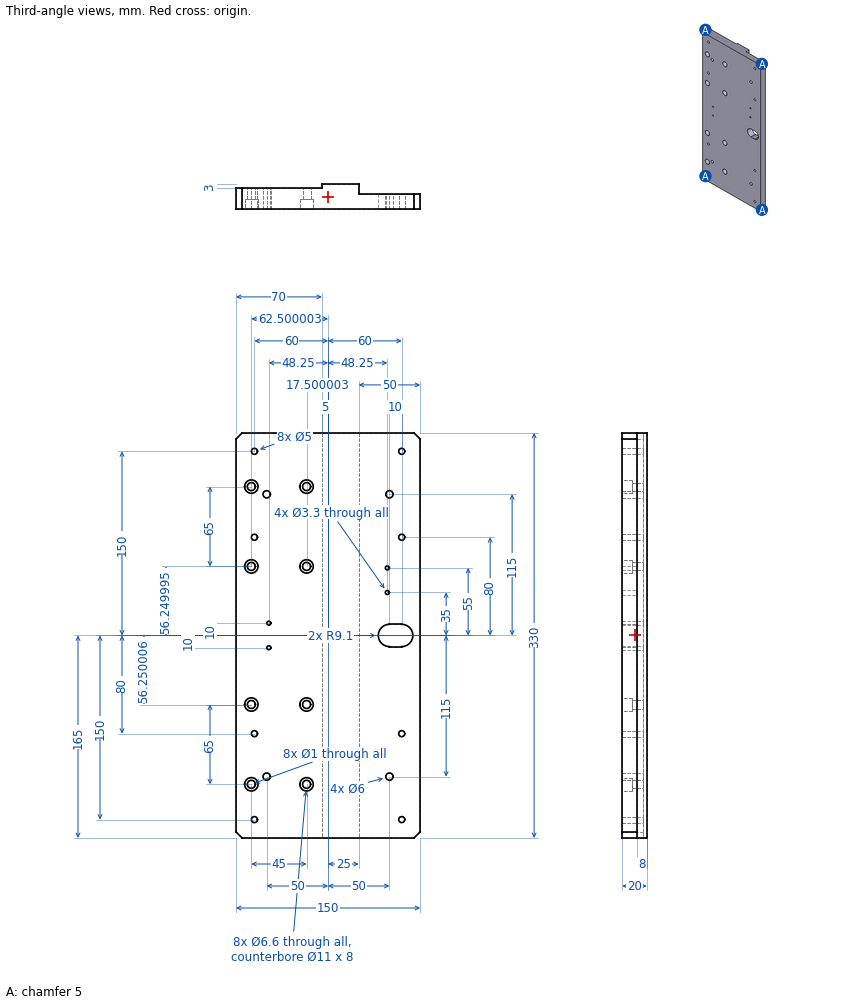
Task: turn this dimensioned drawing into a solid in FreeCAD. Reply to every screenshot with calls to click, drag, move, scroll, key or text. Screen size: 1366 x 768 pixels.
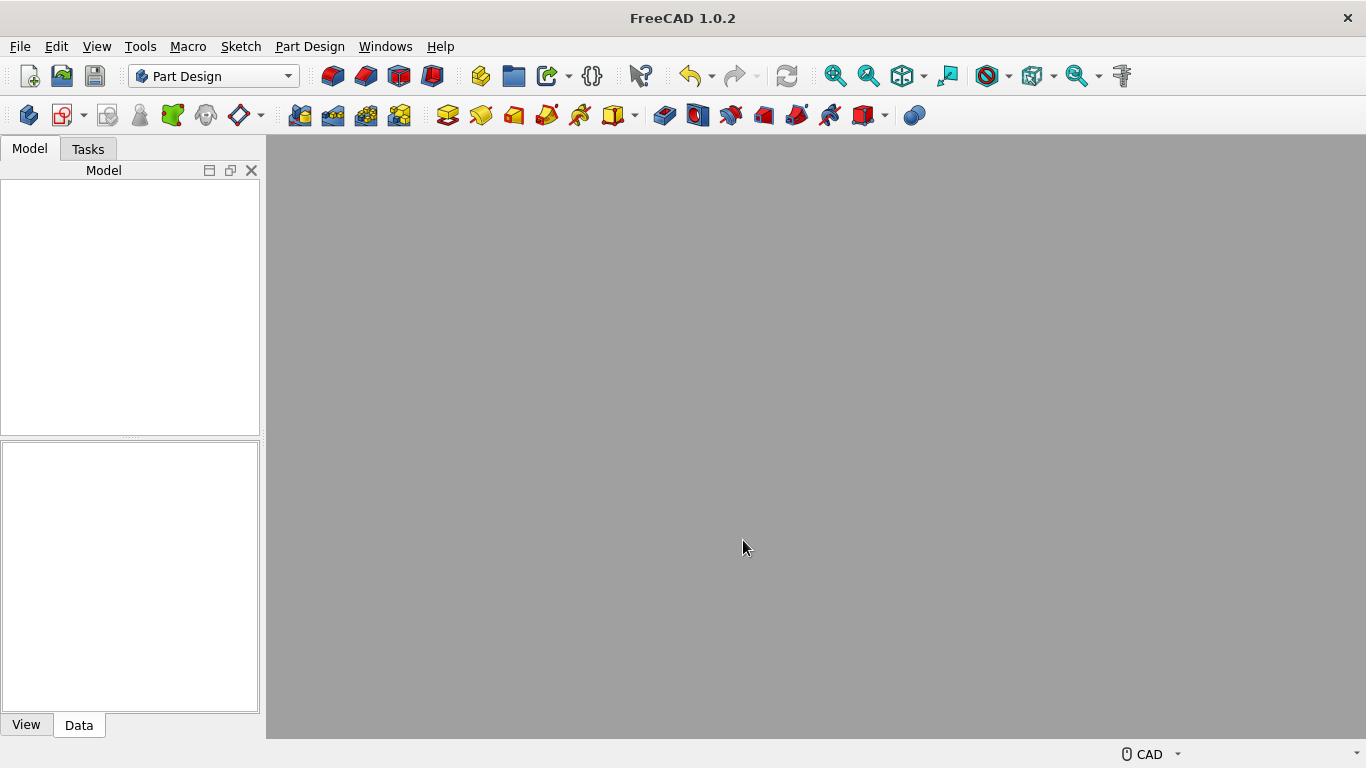
click(29, 76)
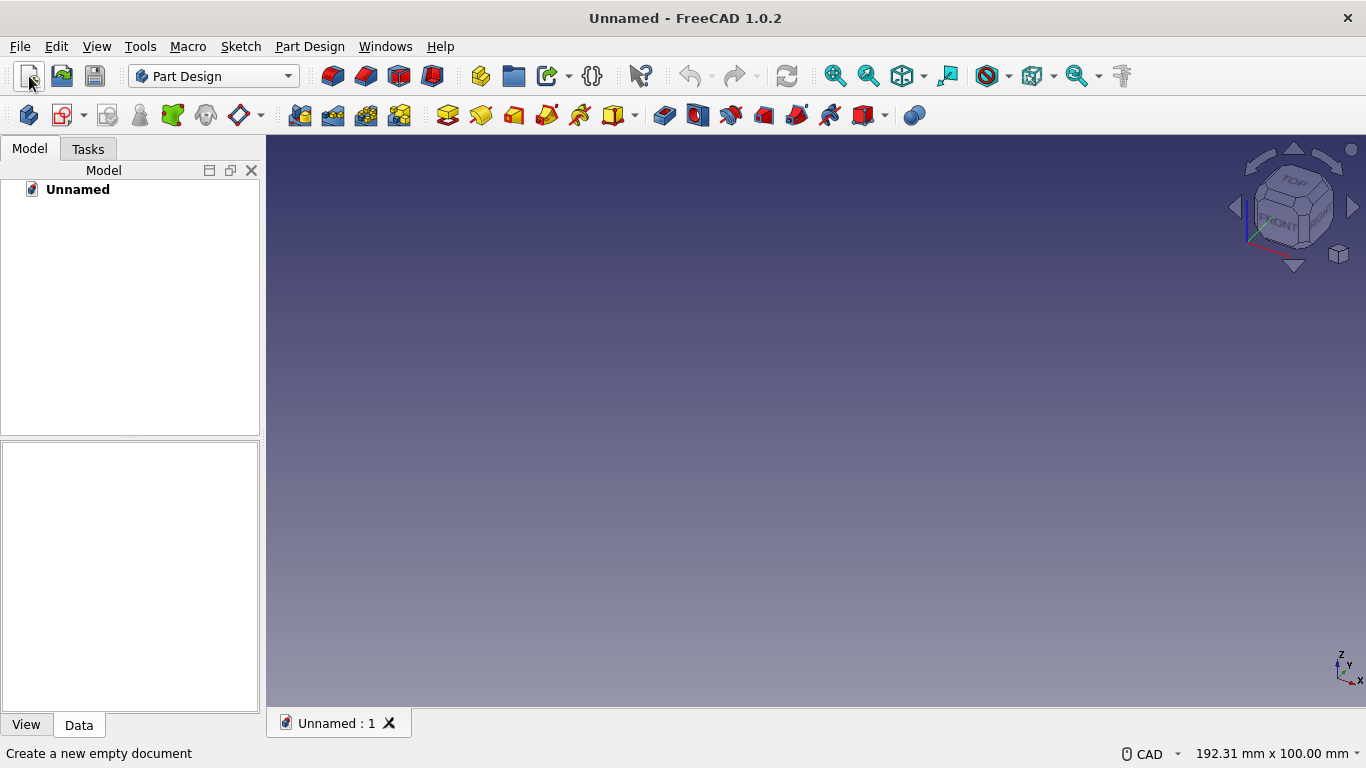
click(62, 116)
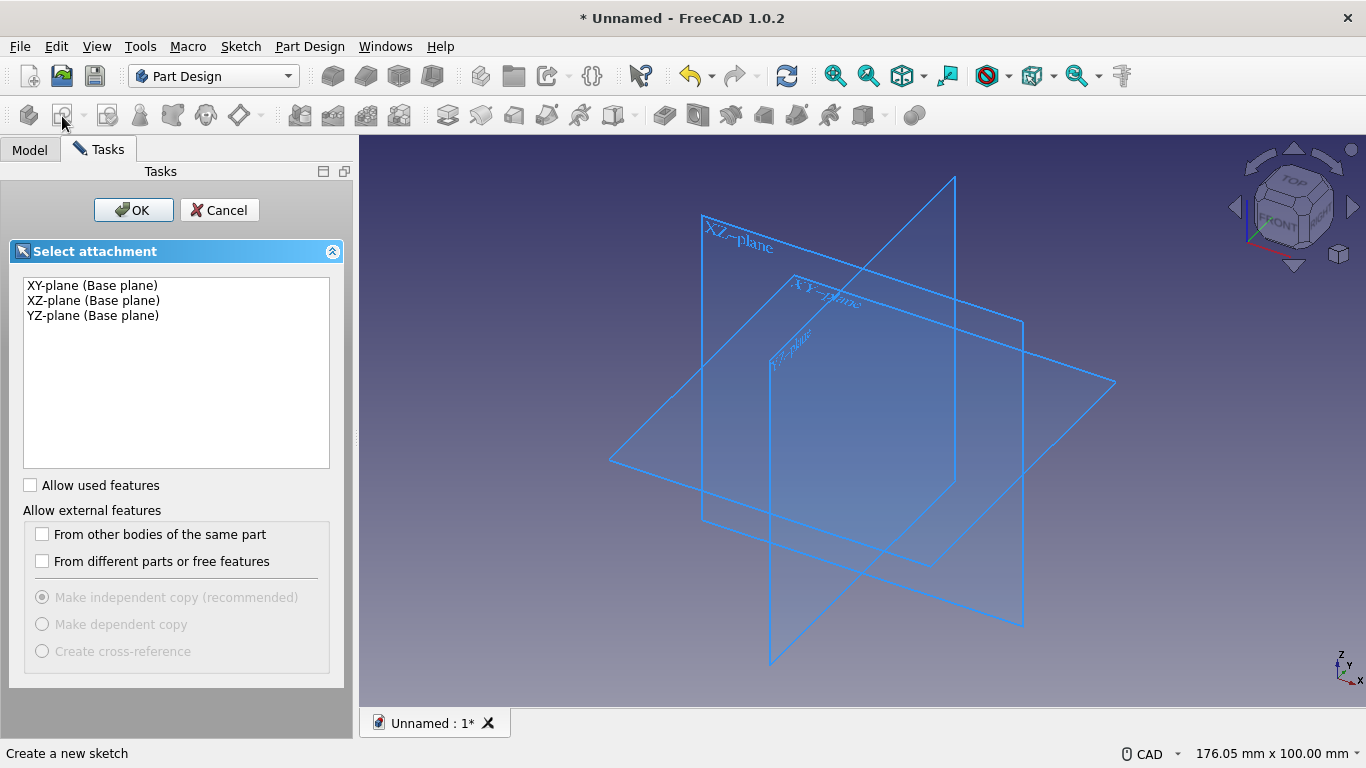
click(84, 300)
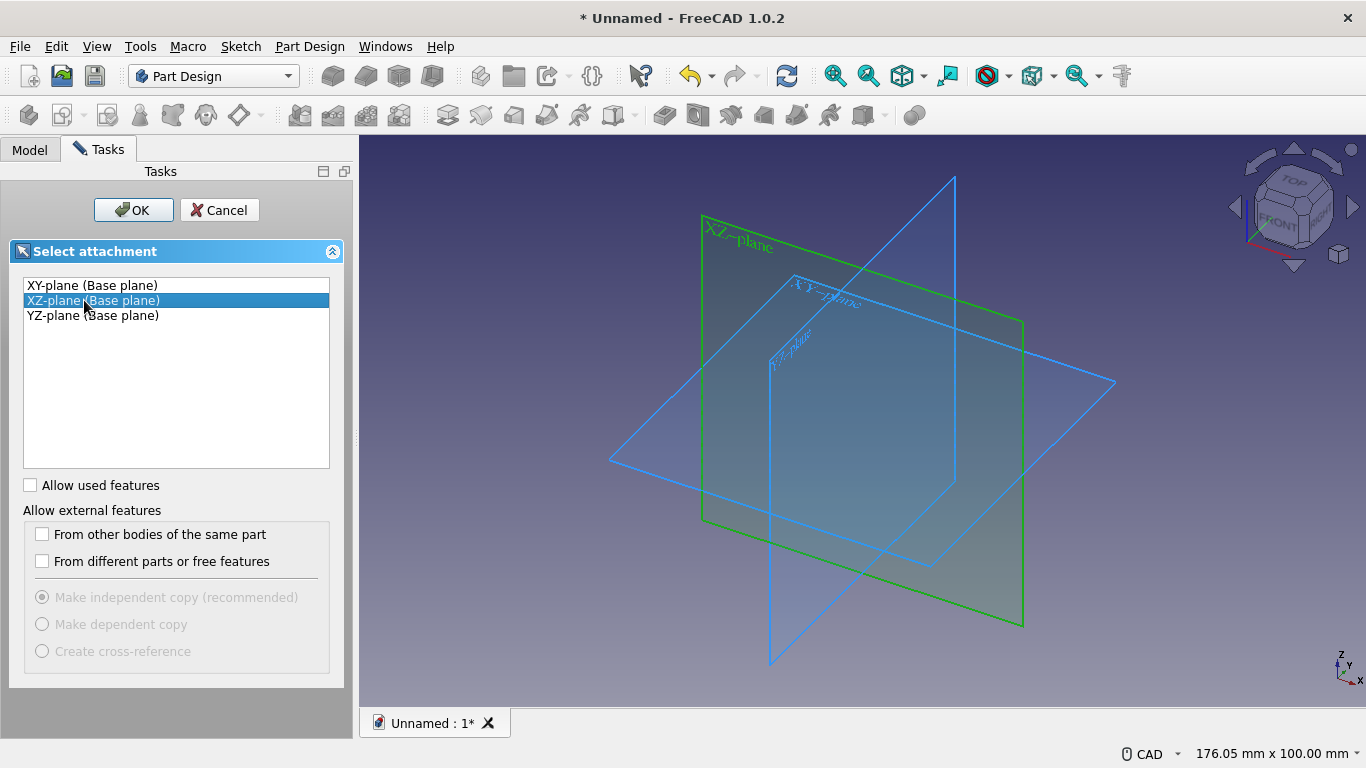
click(134, 210)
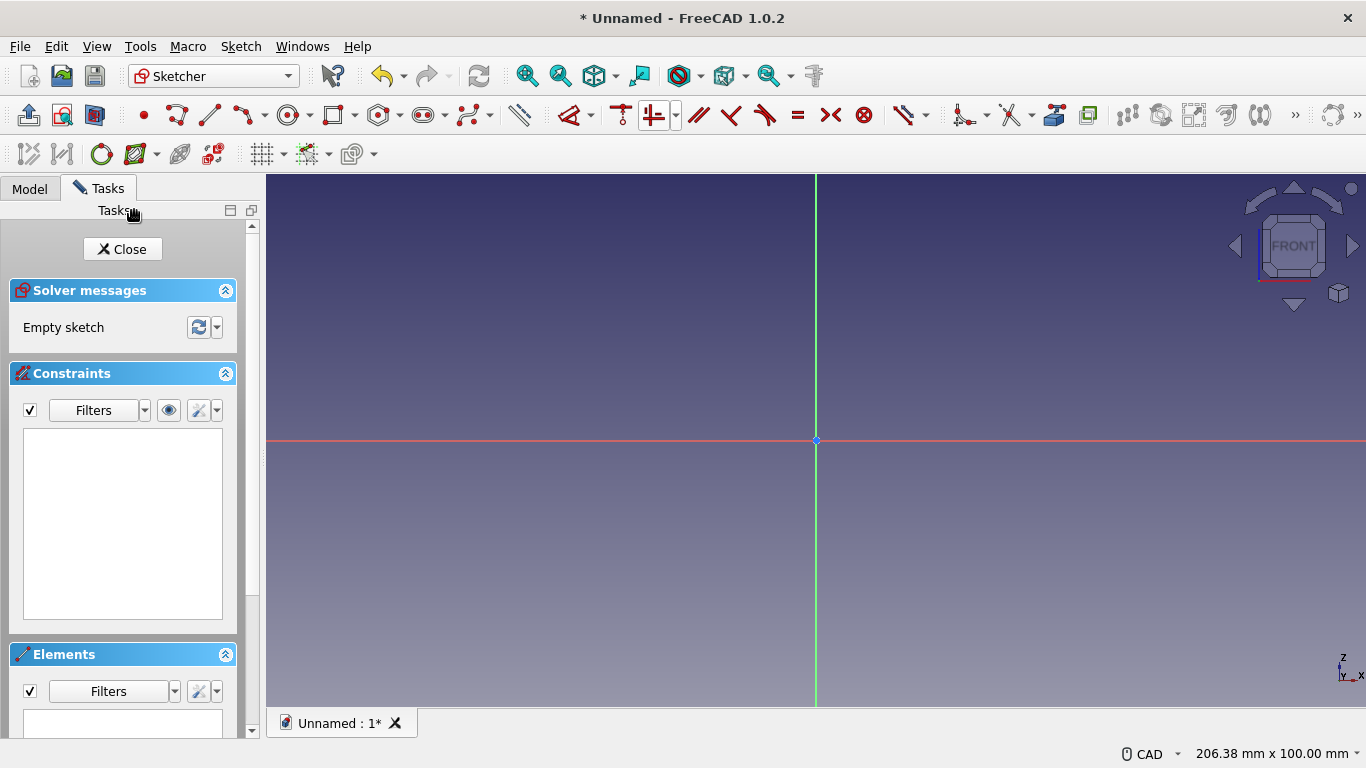
scroll(730, 440, down, 8)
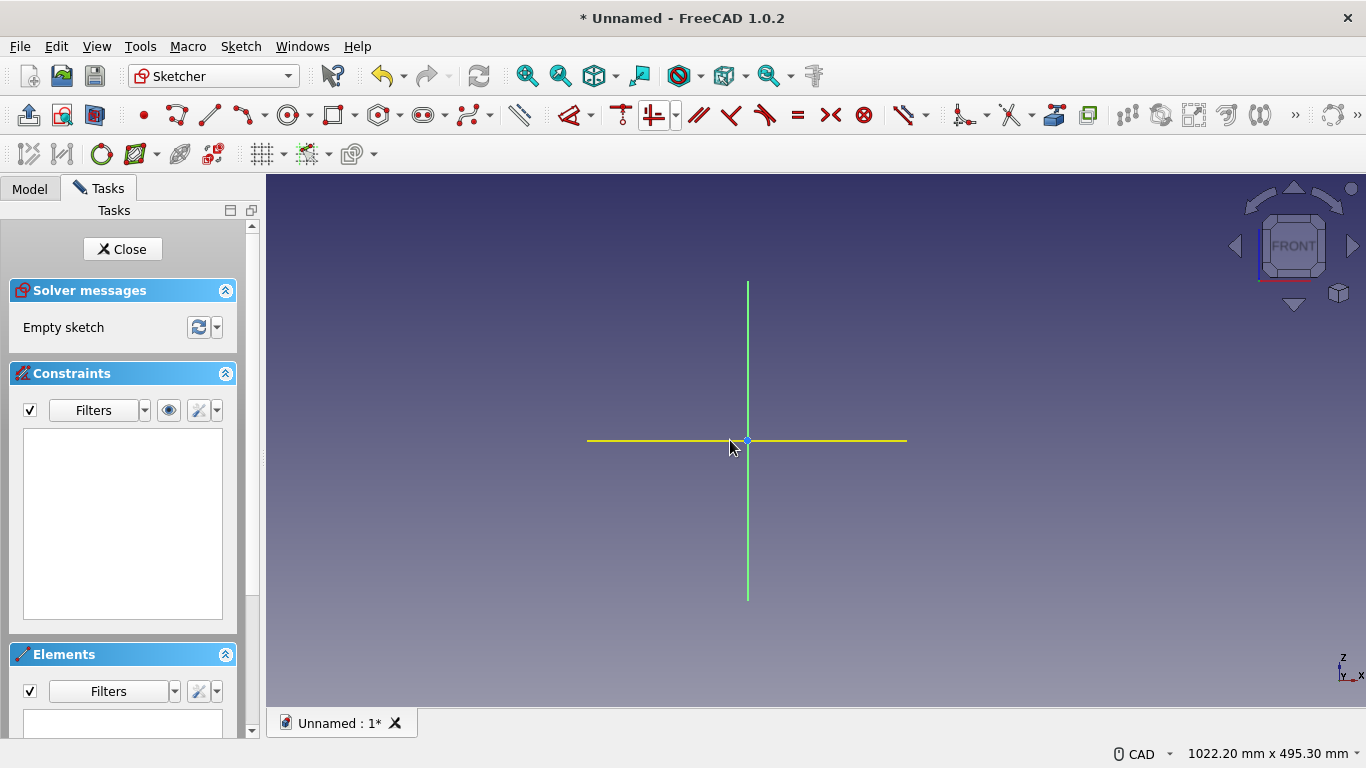
click(354, 116)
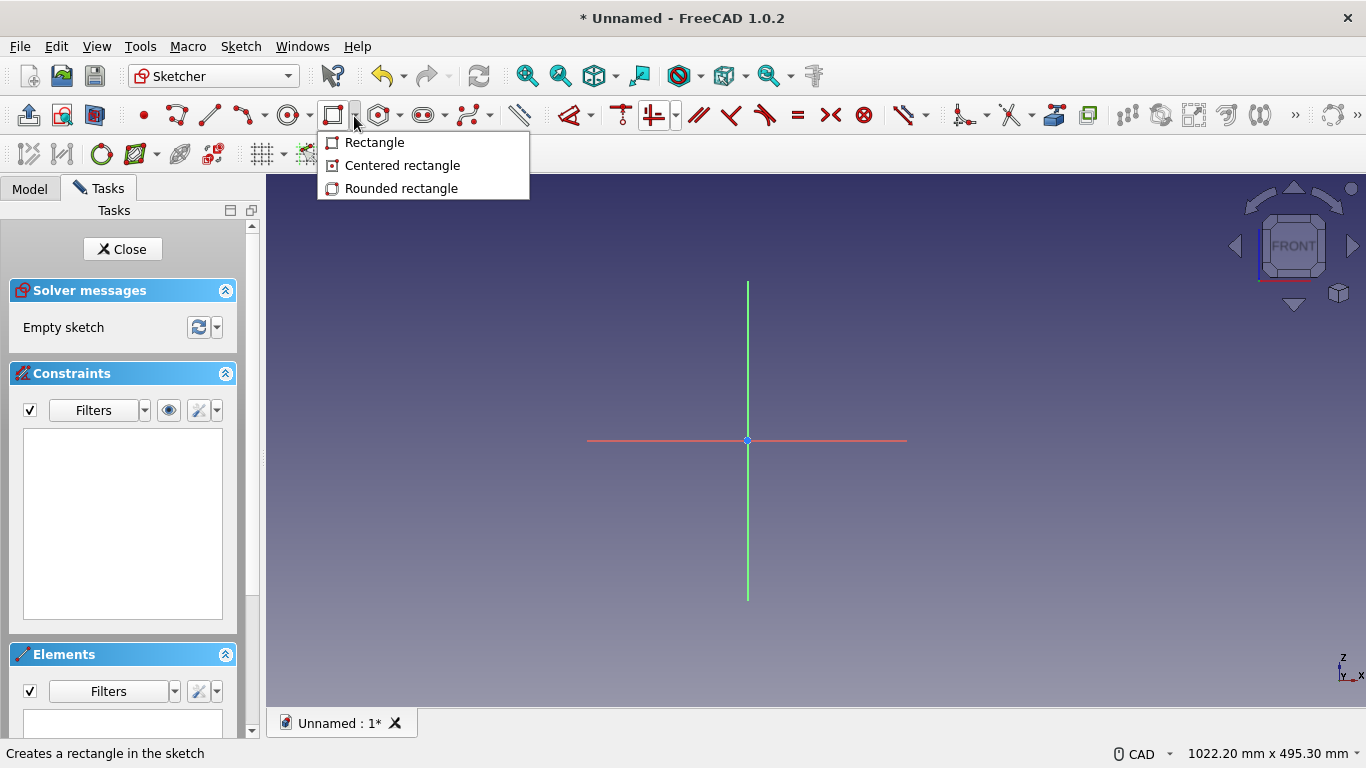
click(424, 166)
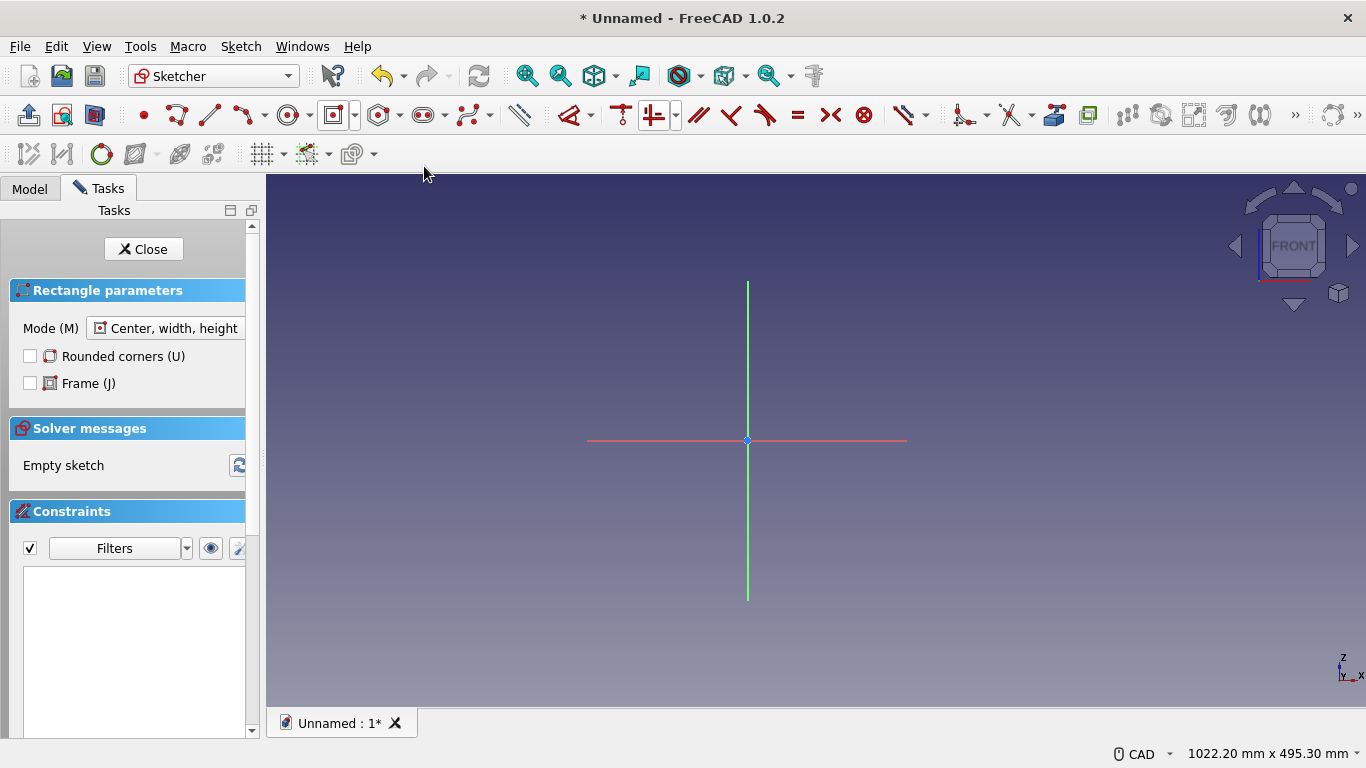
click(748, 440)
move(828, 263)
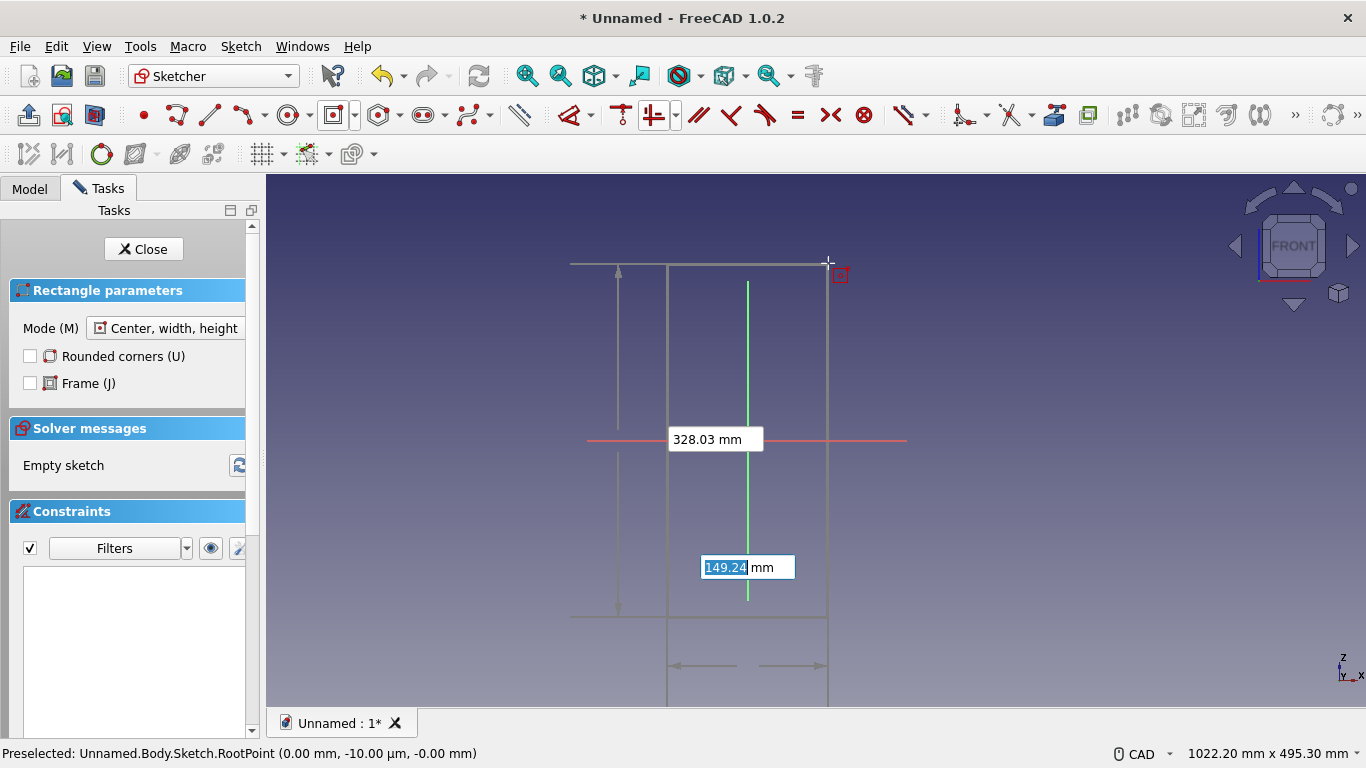
text(150)
key(Tab)
text(330)
key(Return)
key(Escape)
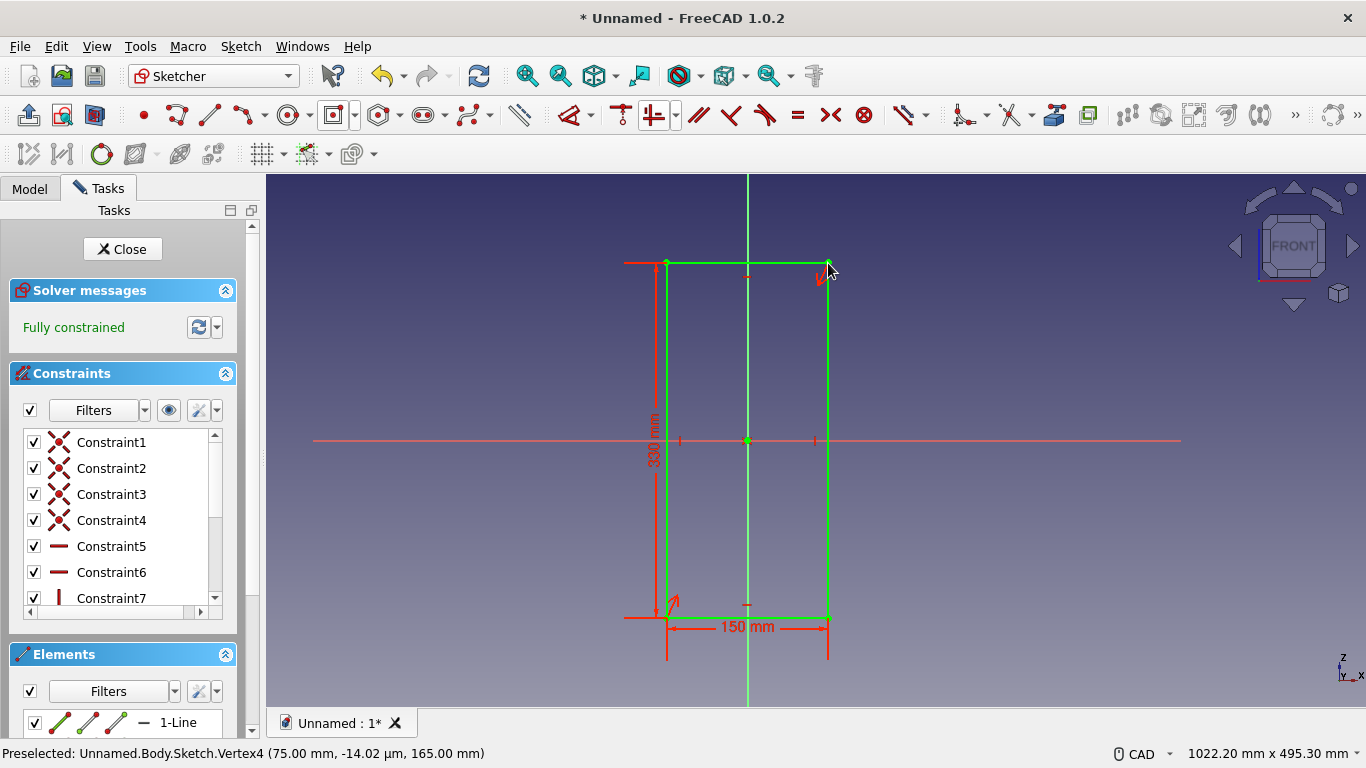
click(123, 249)